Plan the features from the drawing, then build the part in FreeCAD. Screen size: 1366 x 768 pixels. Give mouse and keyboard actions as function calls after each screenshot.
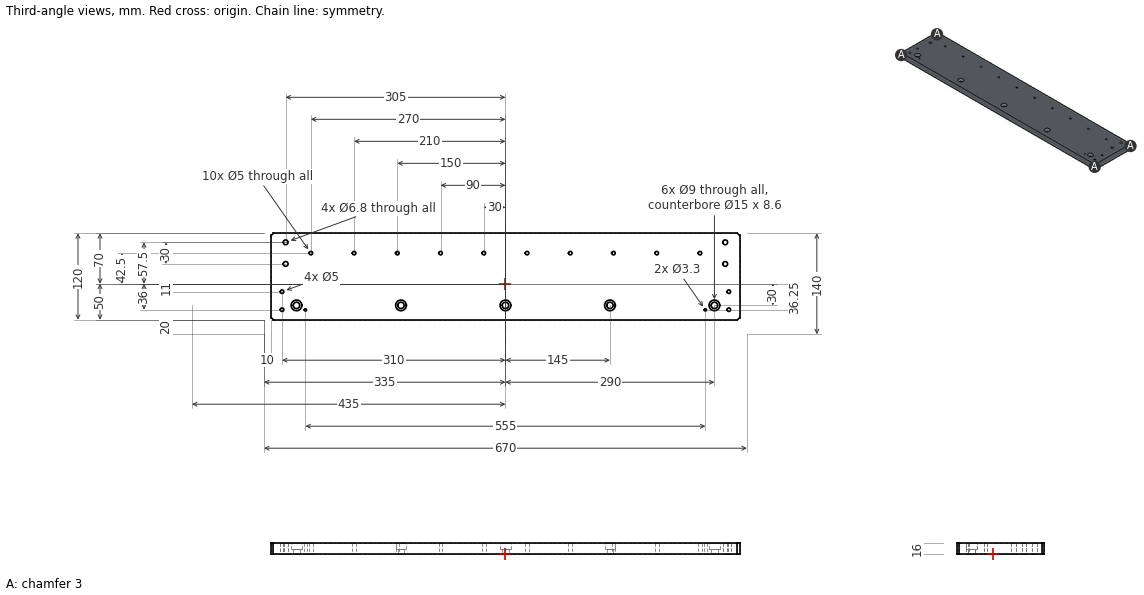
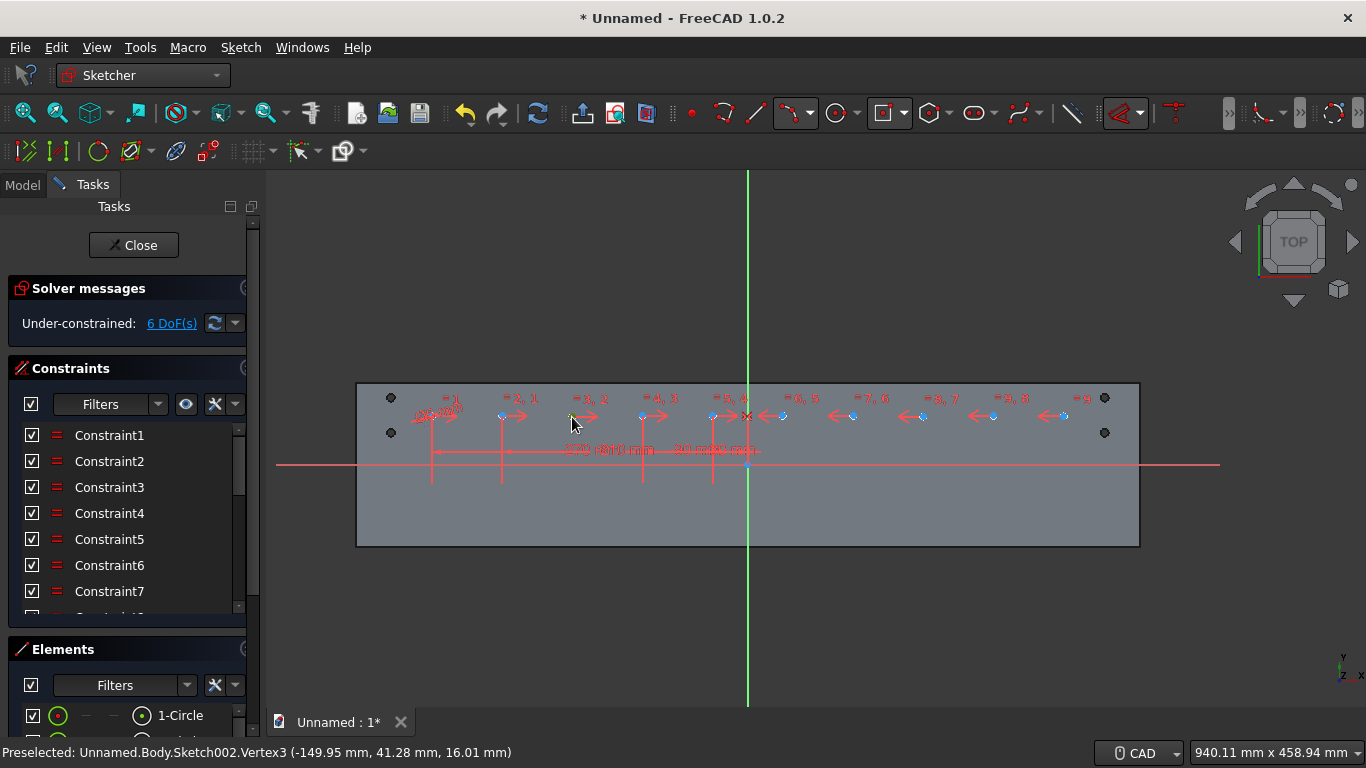
click(1142, 114)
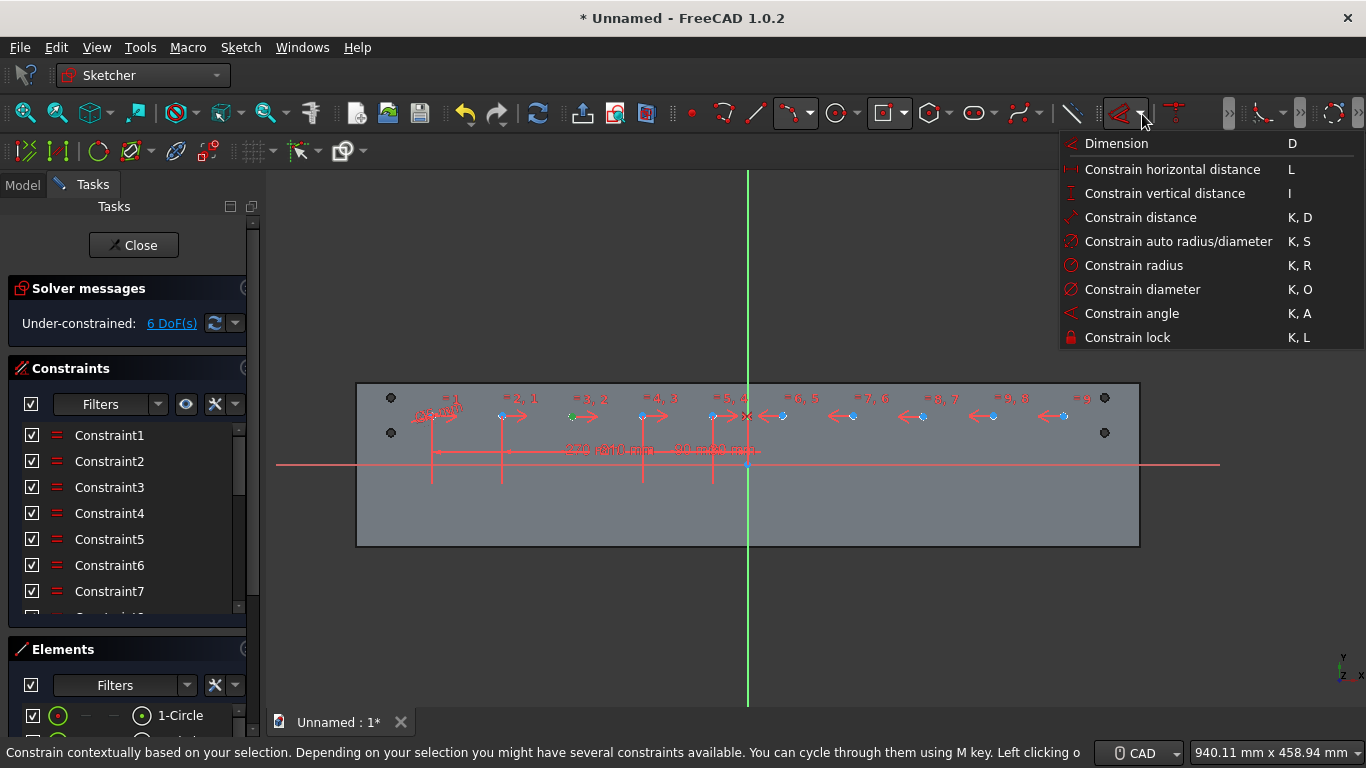
click(1212, 169)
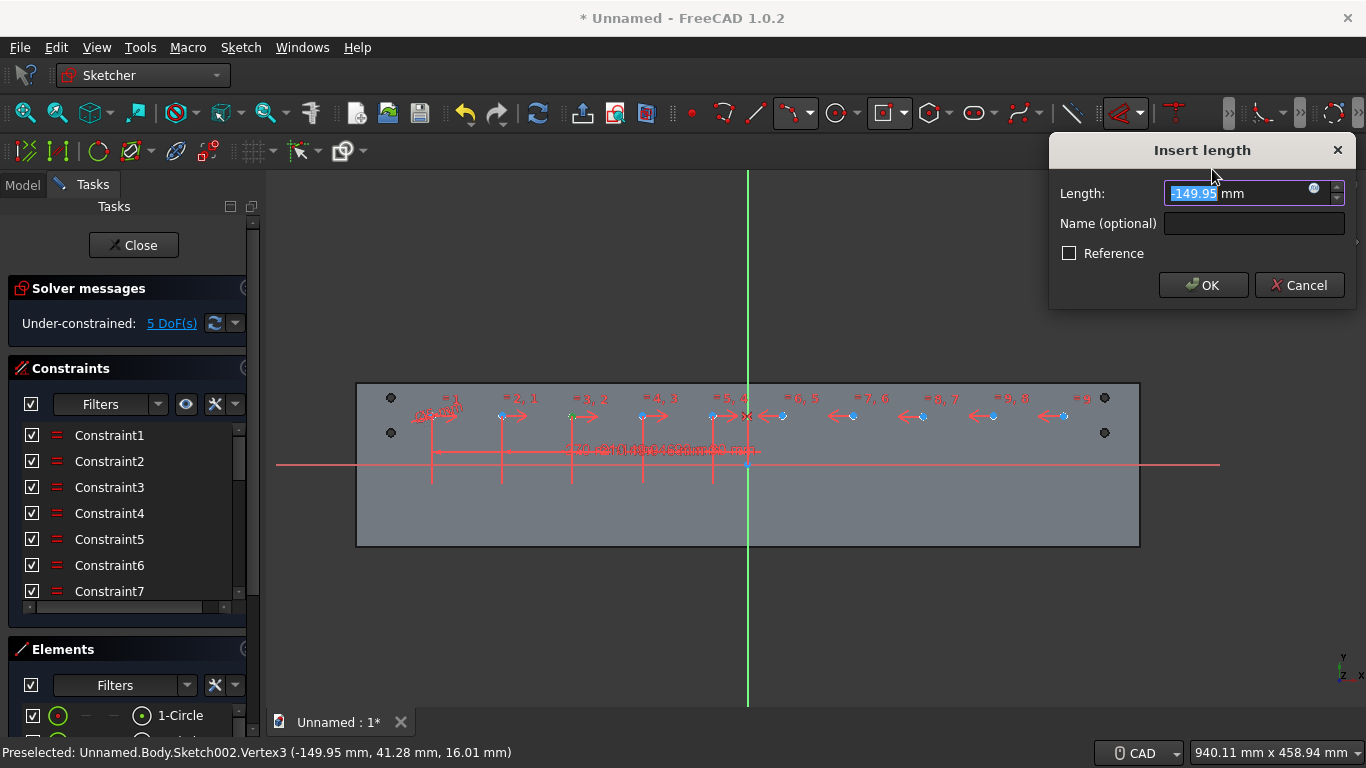
text(-150)
key(Return)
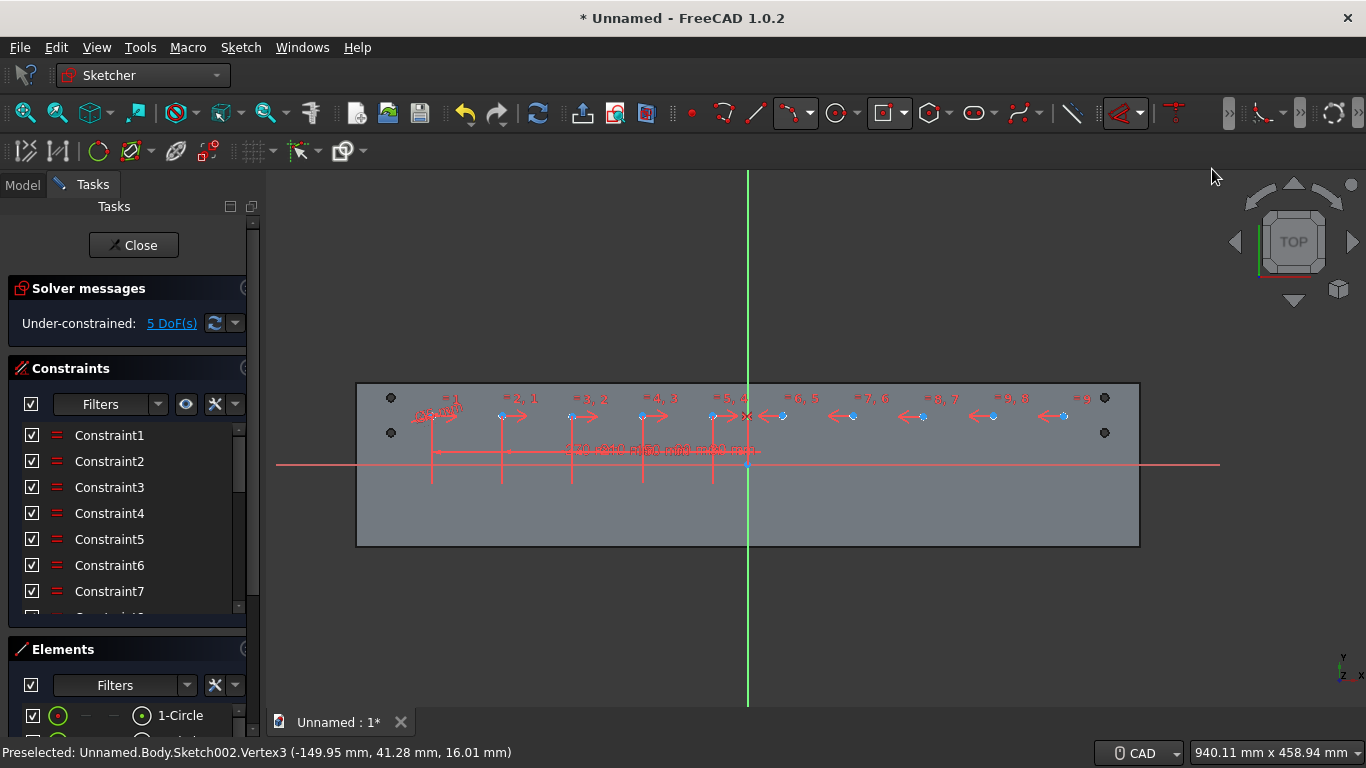
click(432, 416)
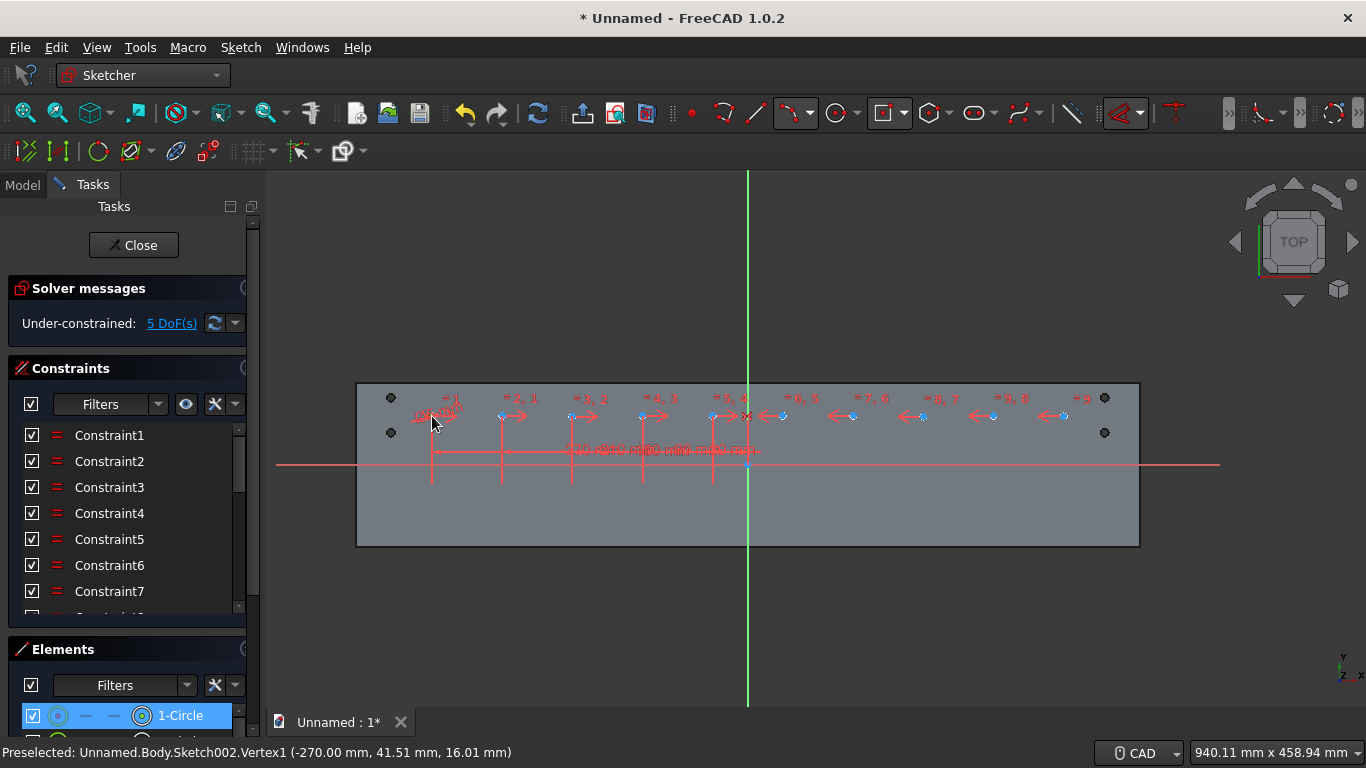
click(1142, 114)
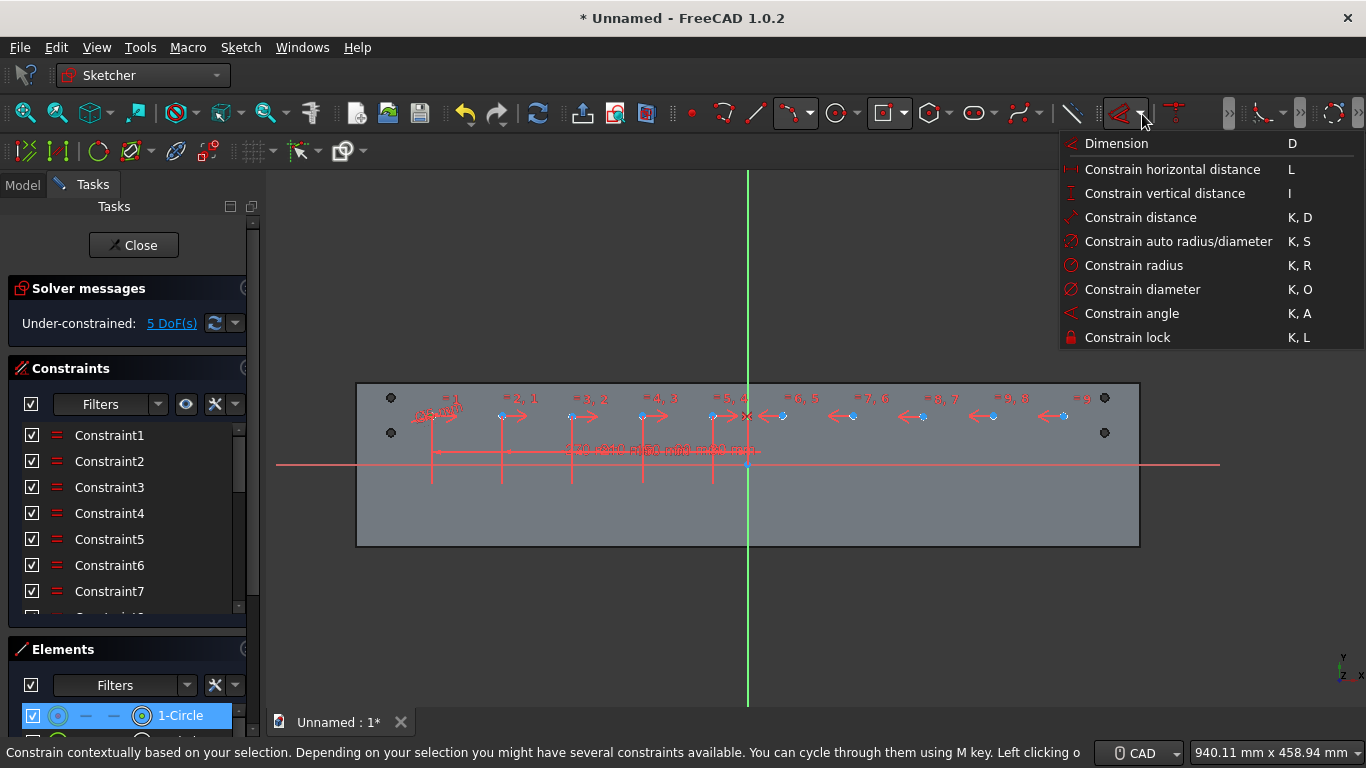
click(1212, 193)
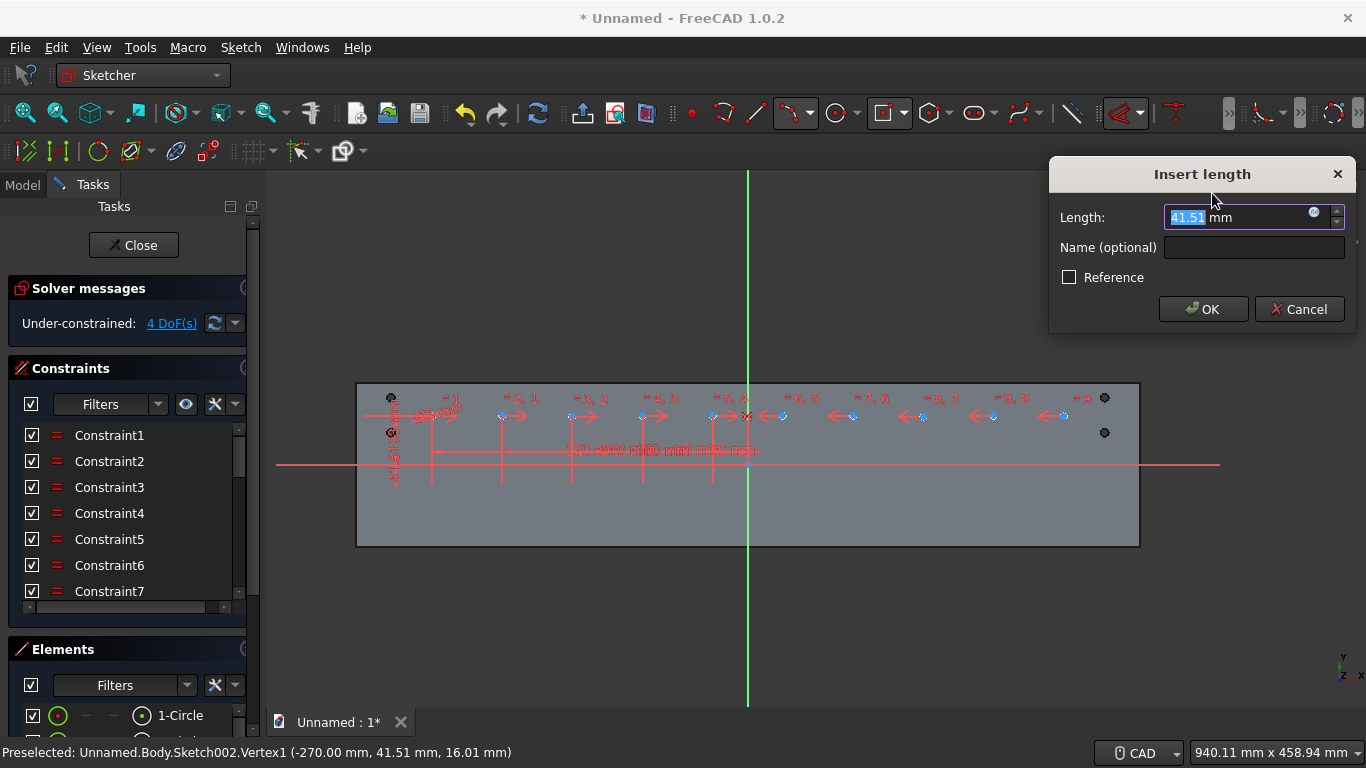
text(42.5)
key(Return)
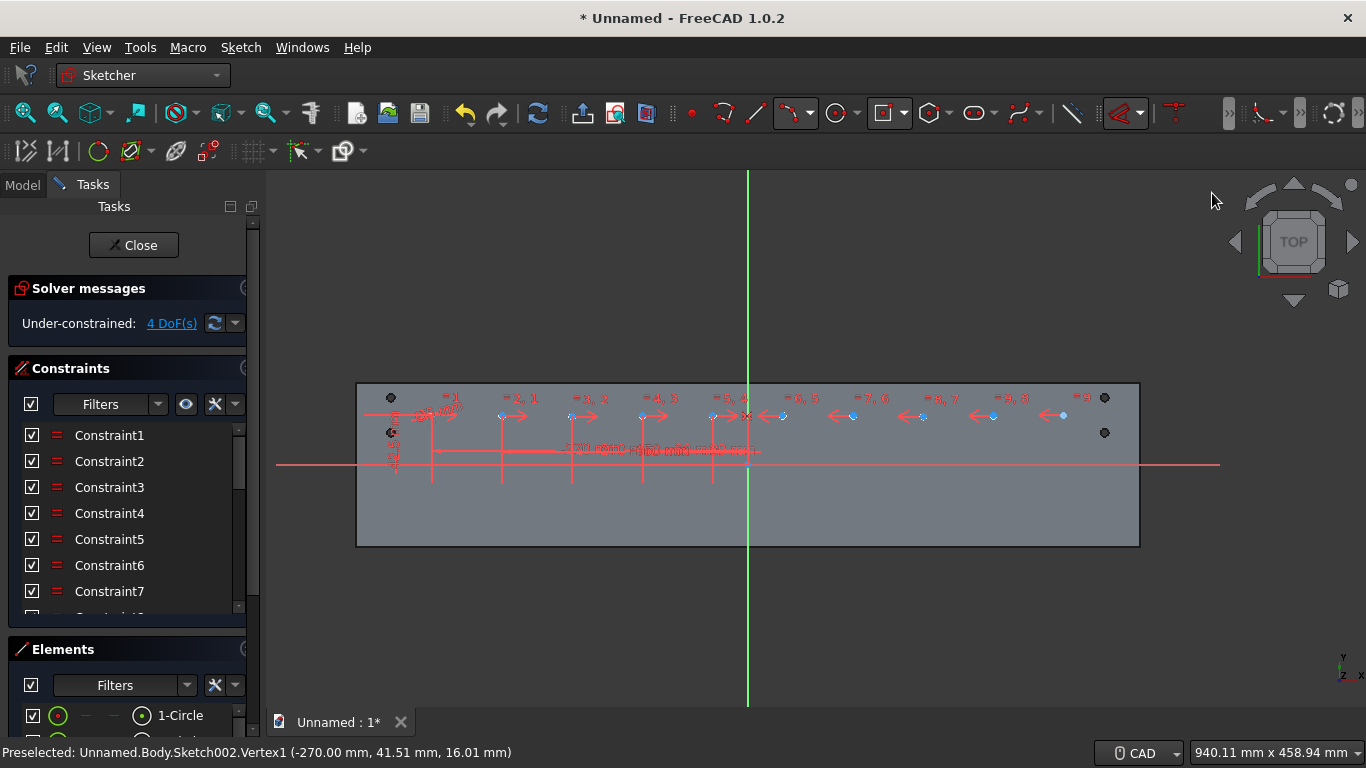
click(502, 416)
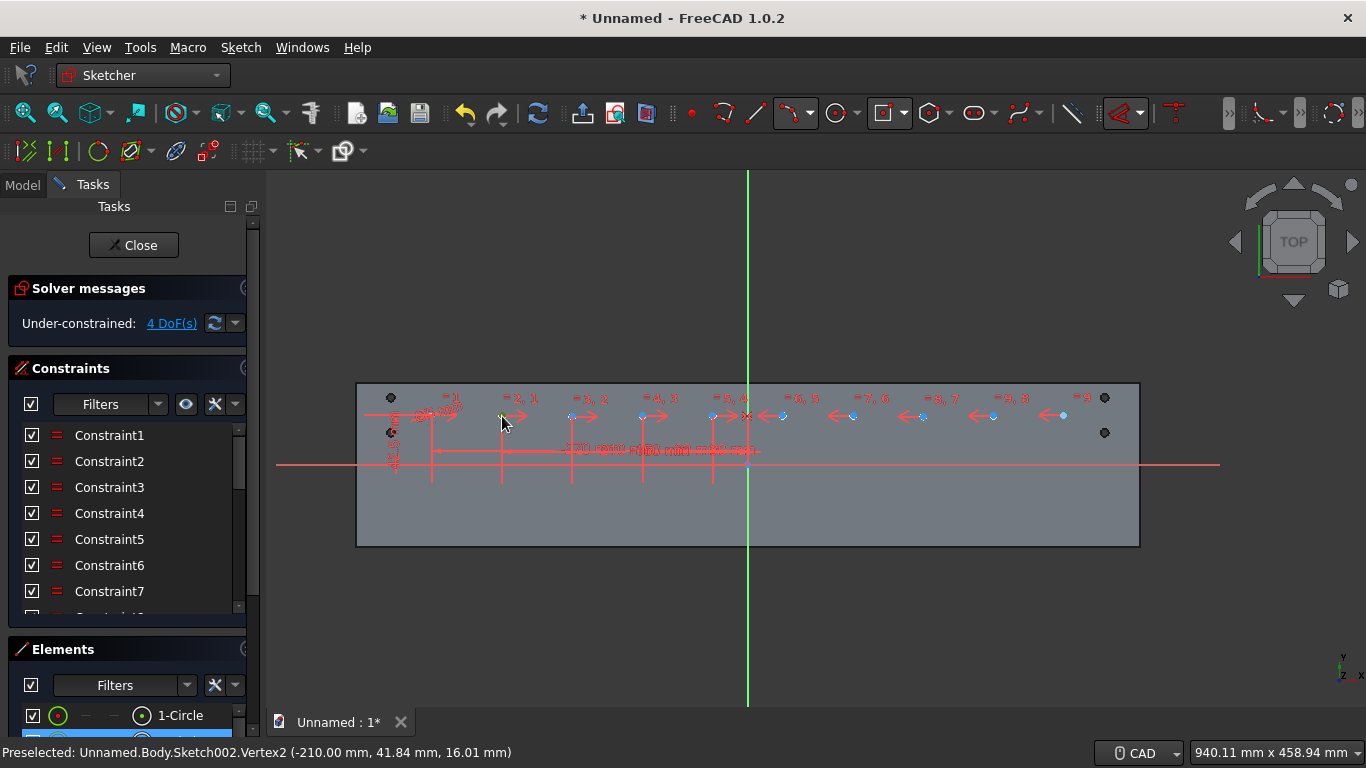
key(i)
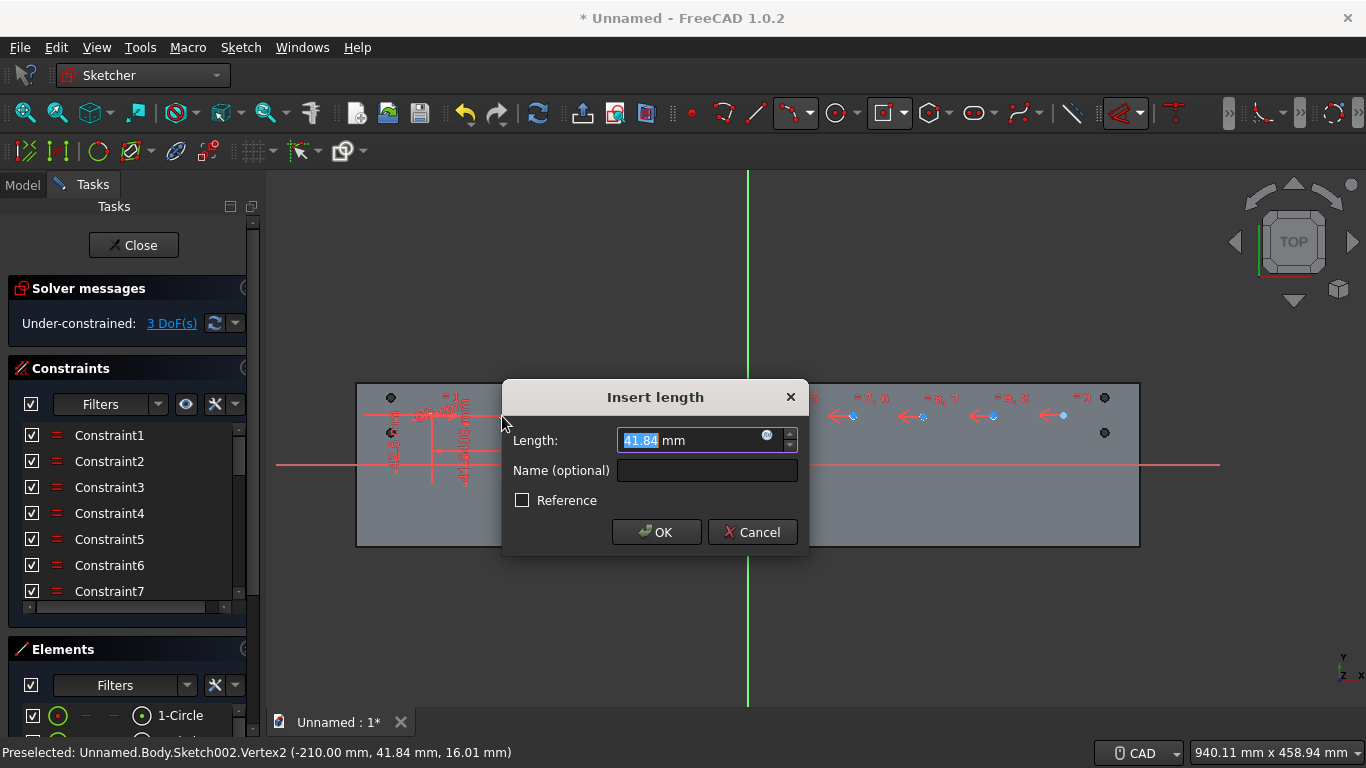
text(42.5)
key(Return)